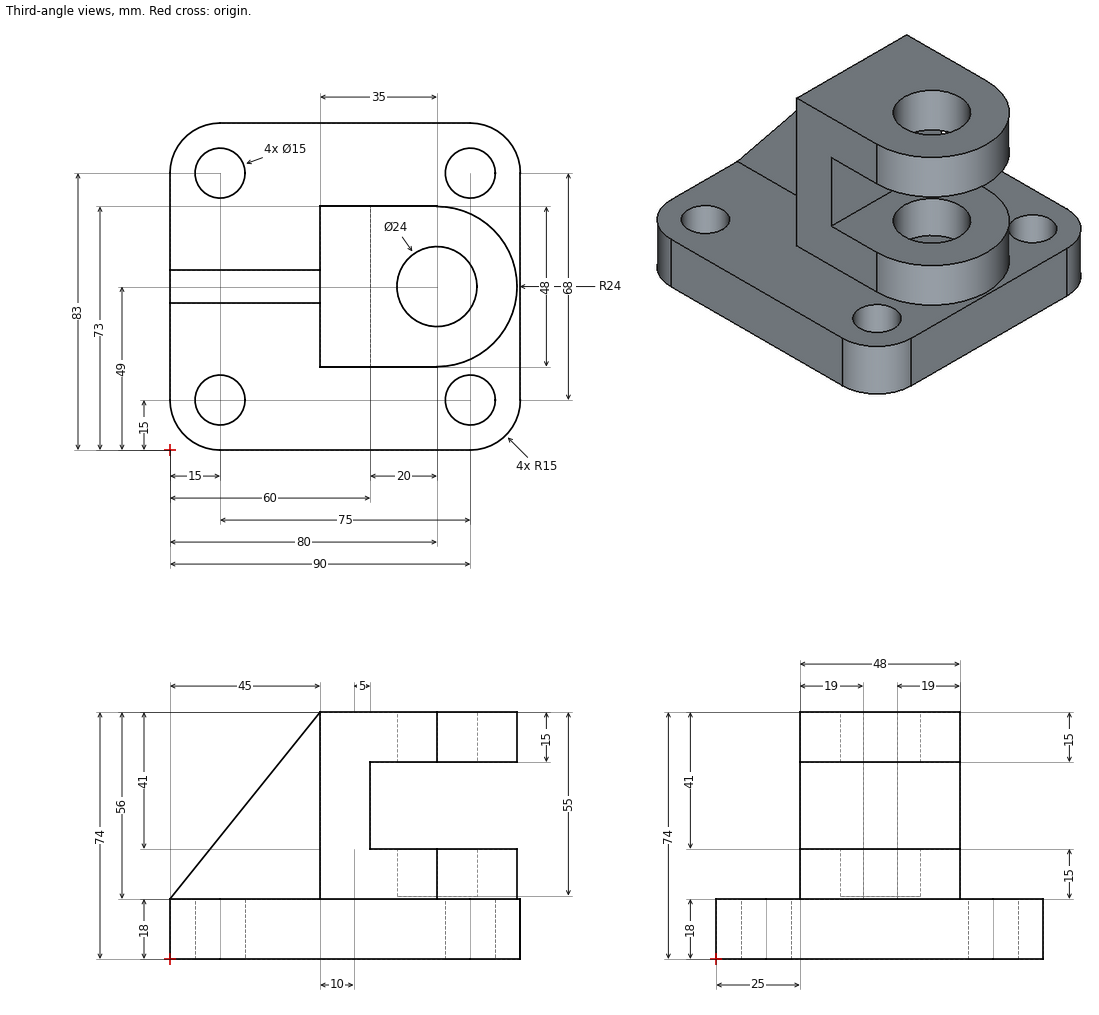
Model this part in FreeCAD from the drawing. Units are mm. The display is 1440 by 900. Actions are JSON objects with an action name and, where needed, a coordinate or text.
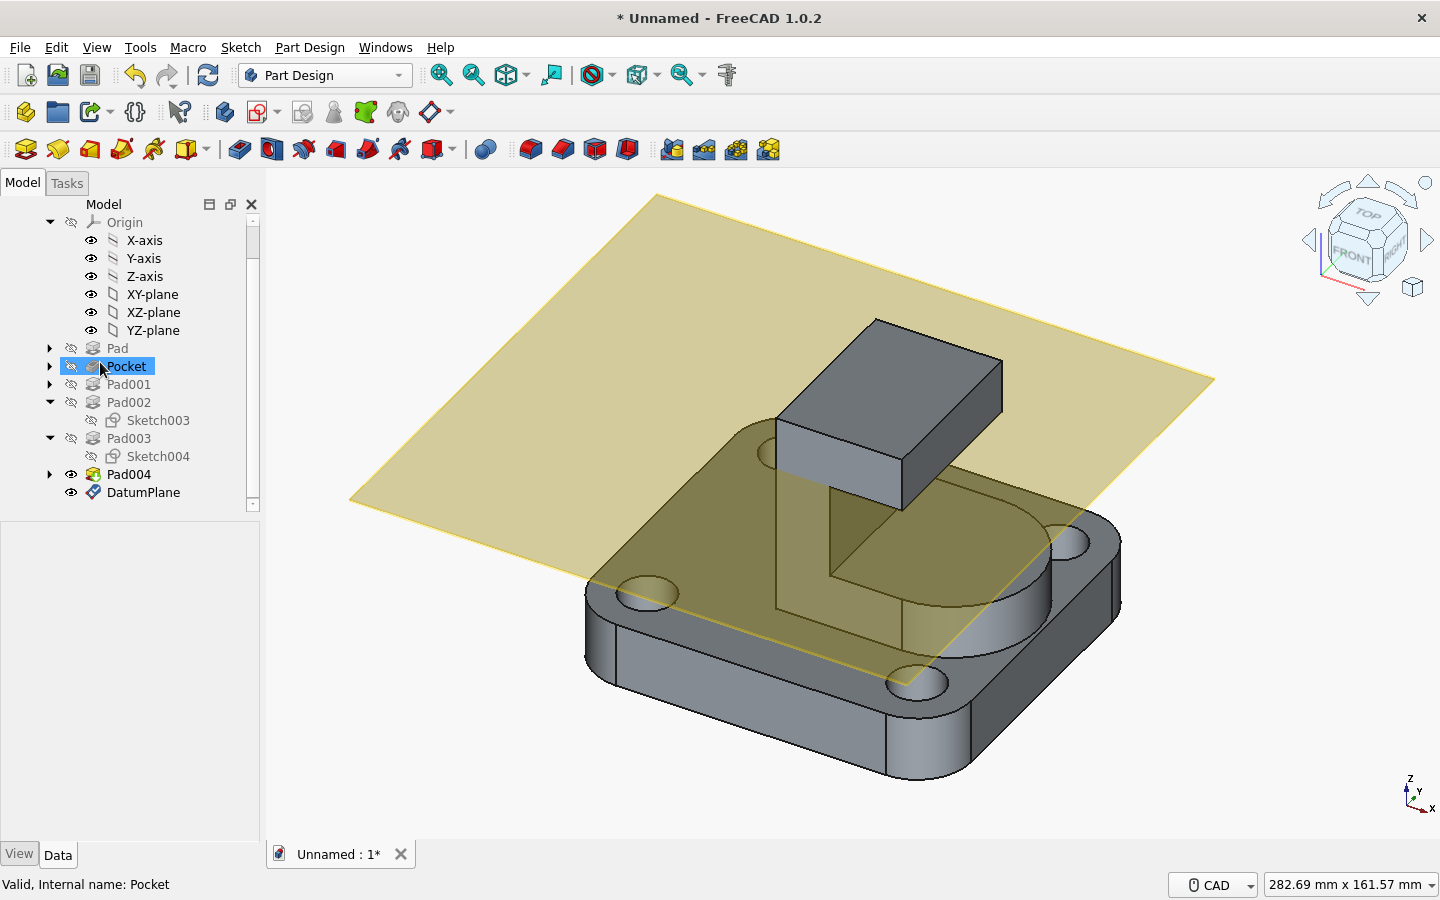
{"action": "left_click", "coordinate": [116, 492]}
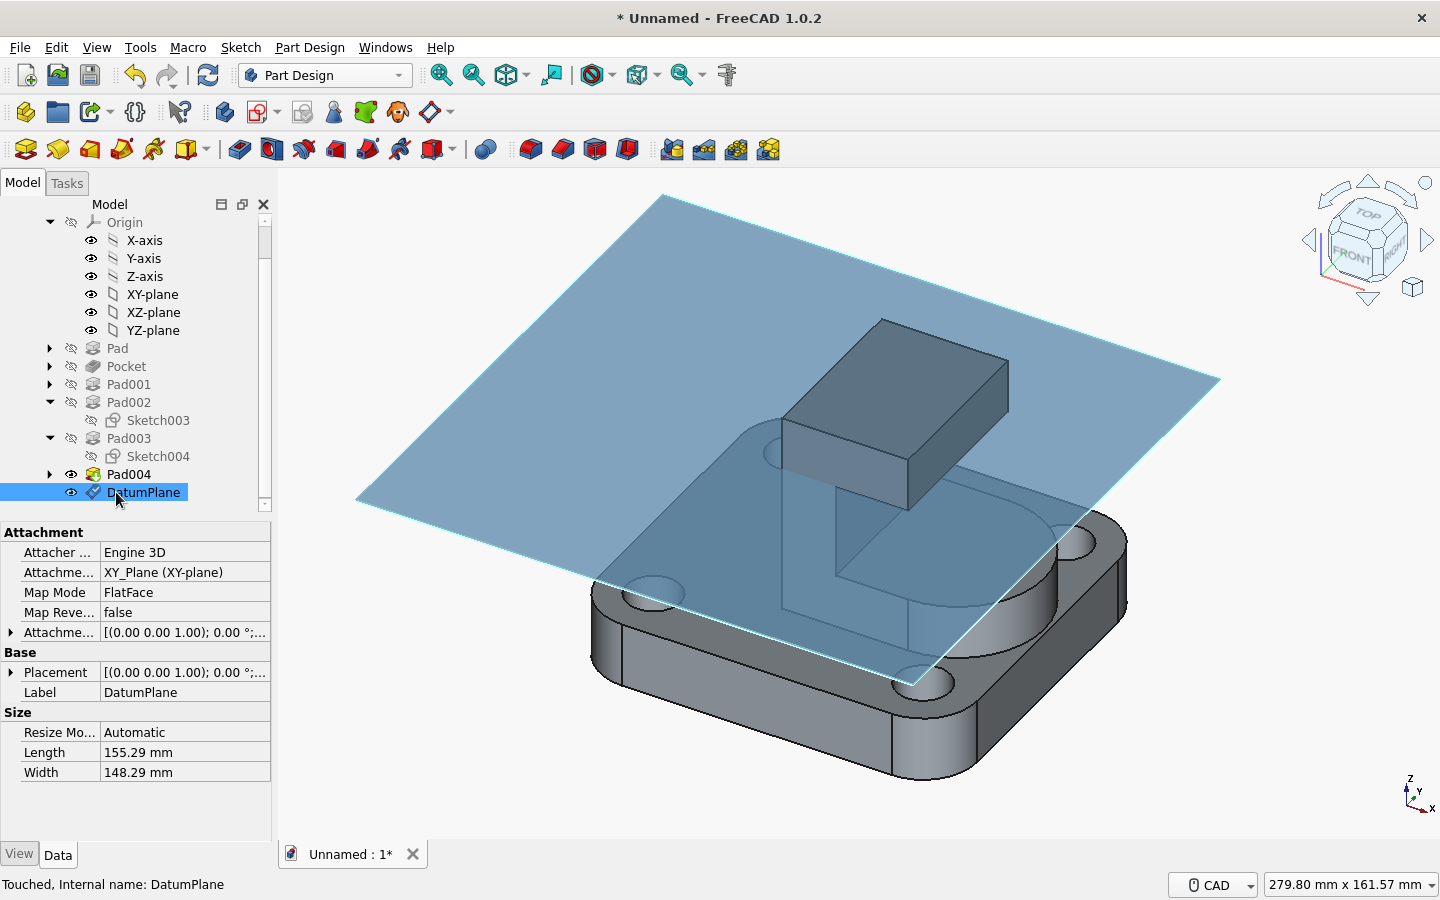
{"action": "left_click", "coordinate": [258, 112]}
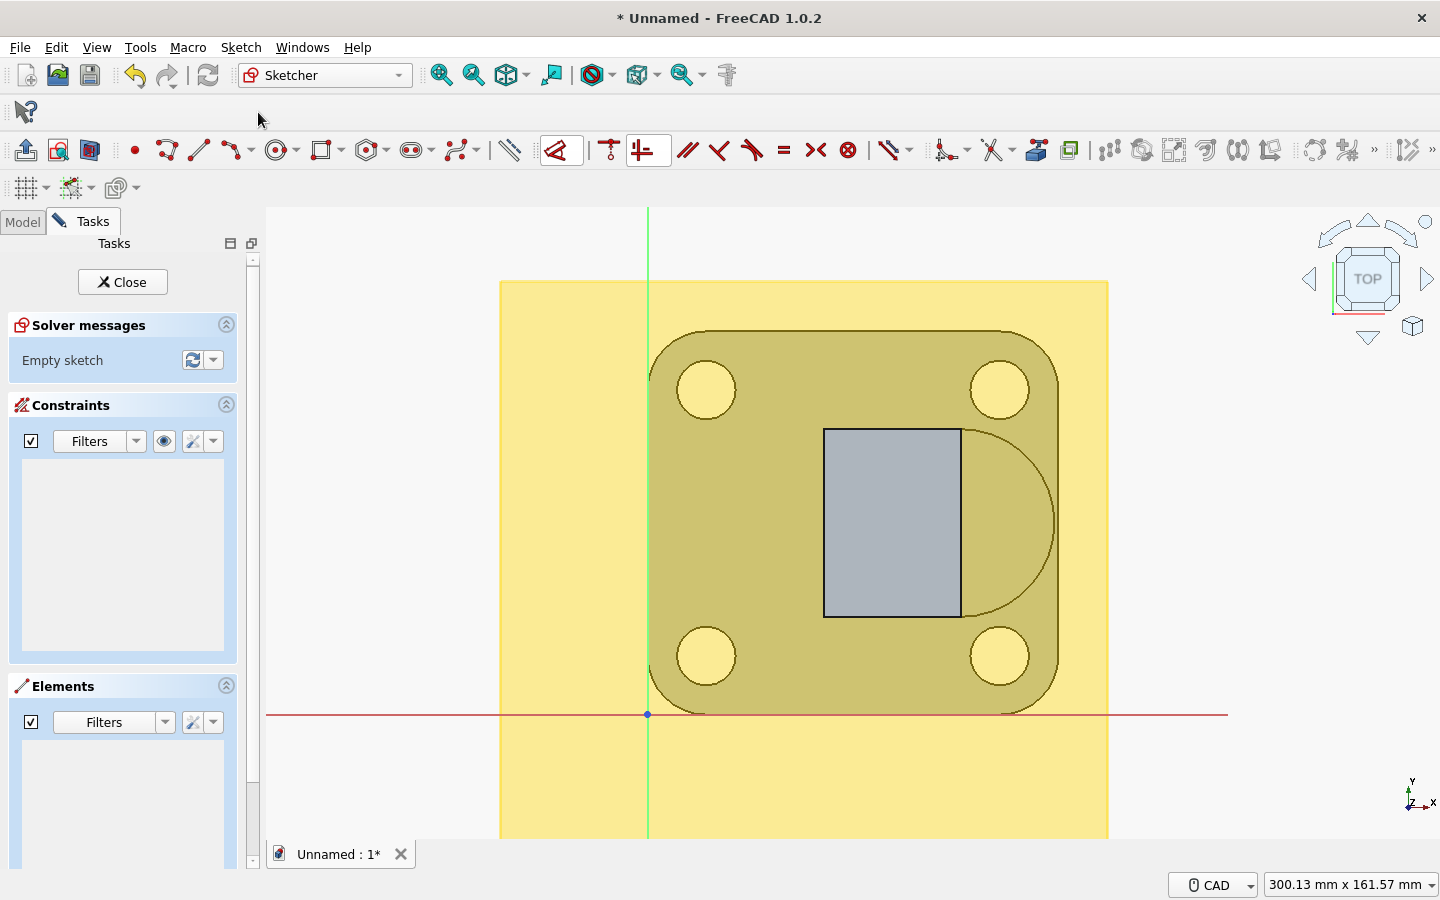
{"action": "left_click", "coordinate": [90, 150]}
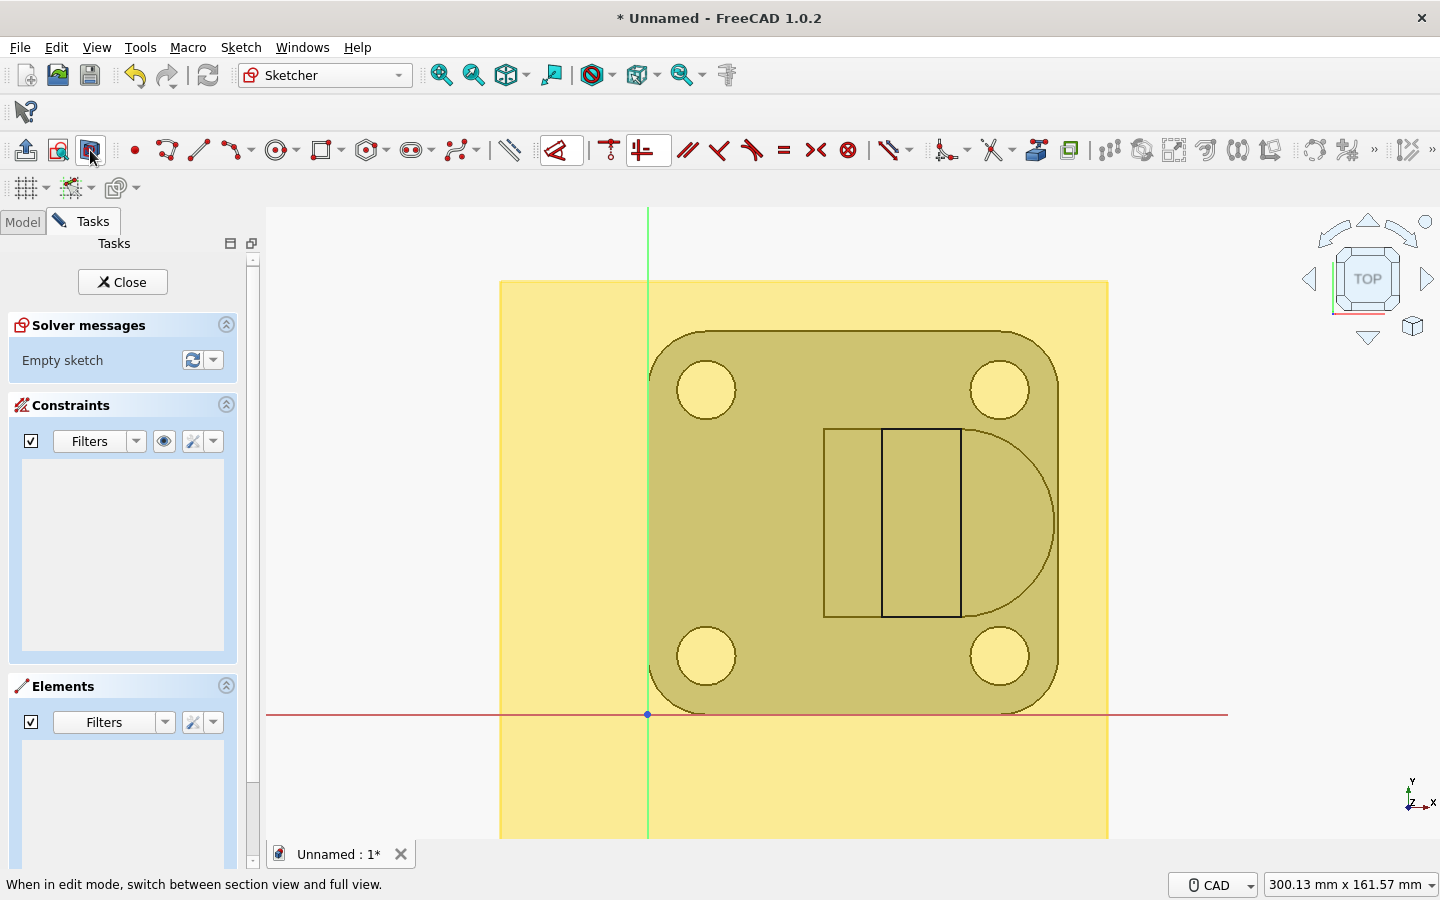
{"action": "scroll", "coordinate": [986, 671], "scroll_direction": "up", "scroll_amount": 2}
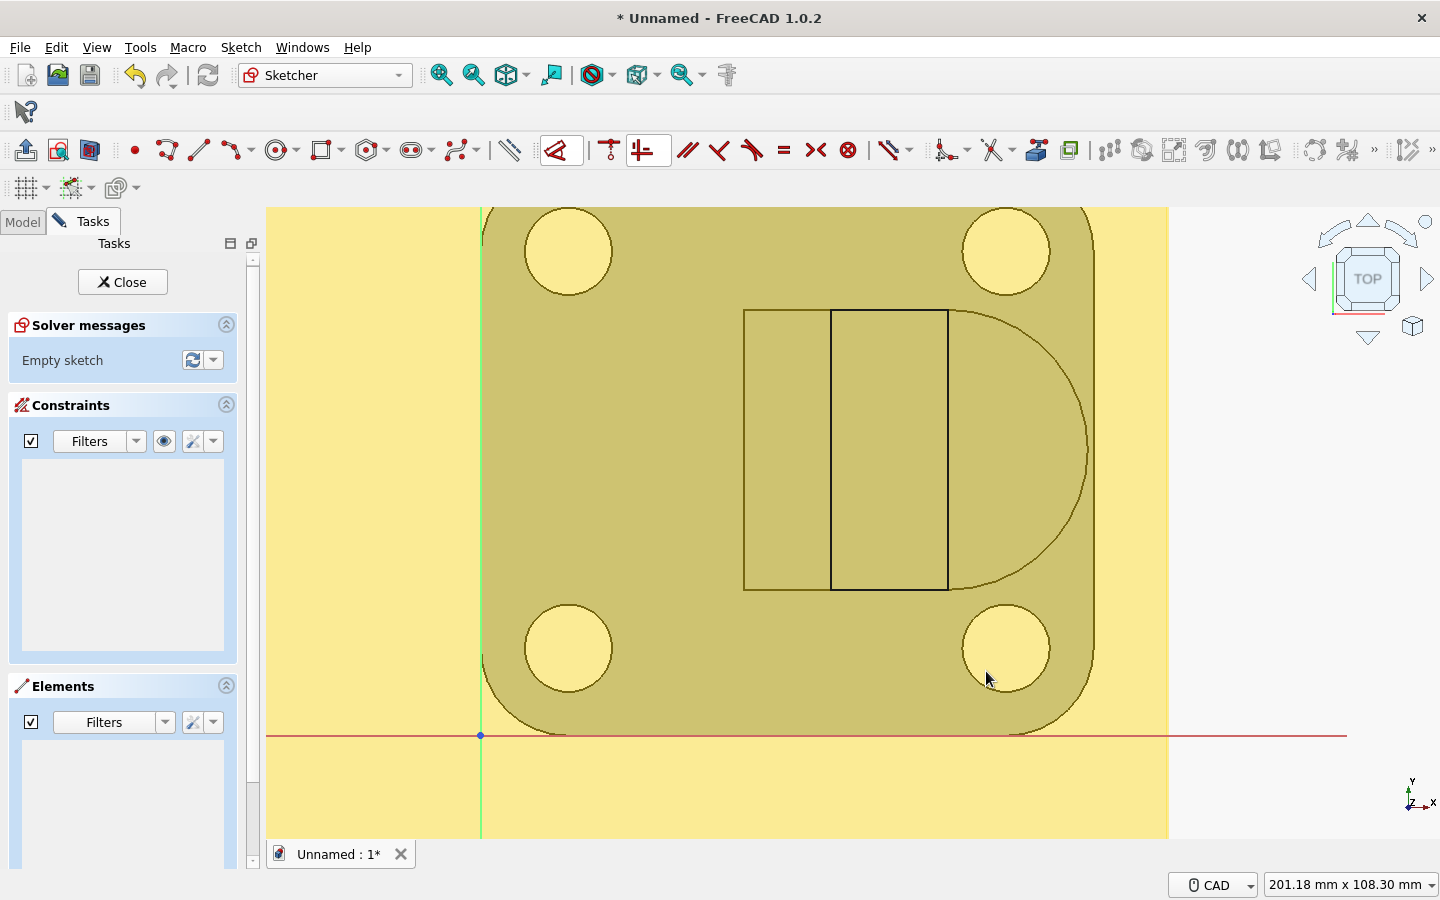
{"action": "left_click", "coordinate": [200, 150]}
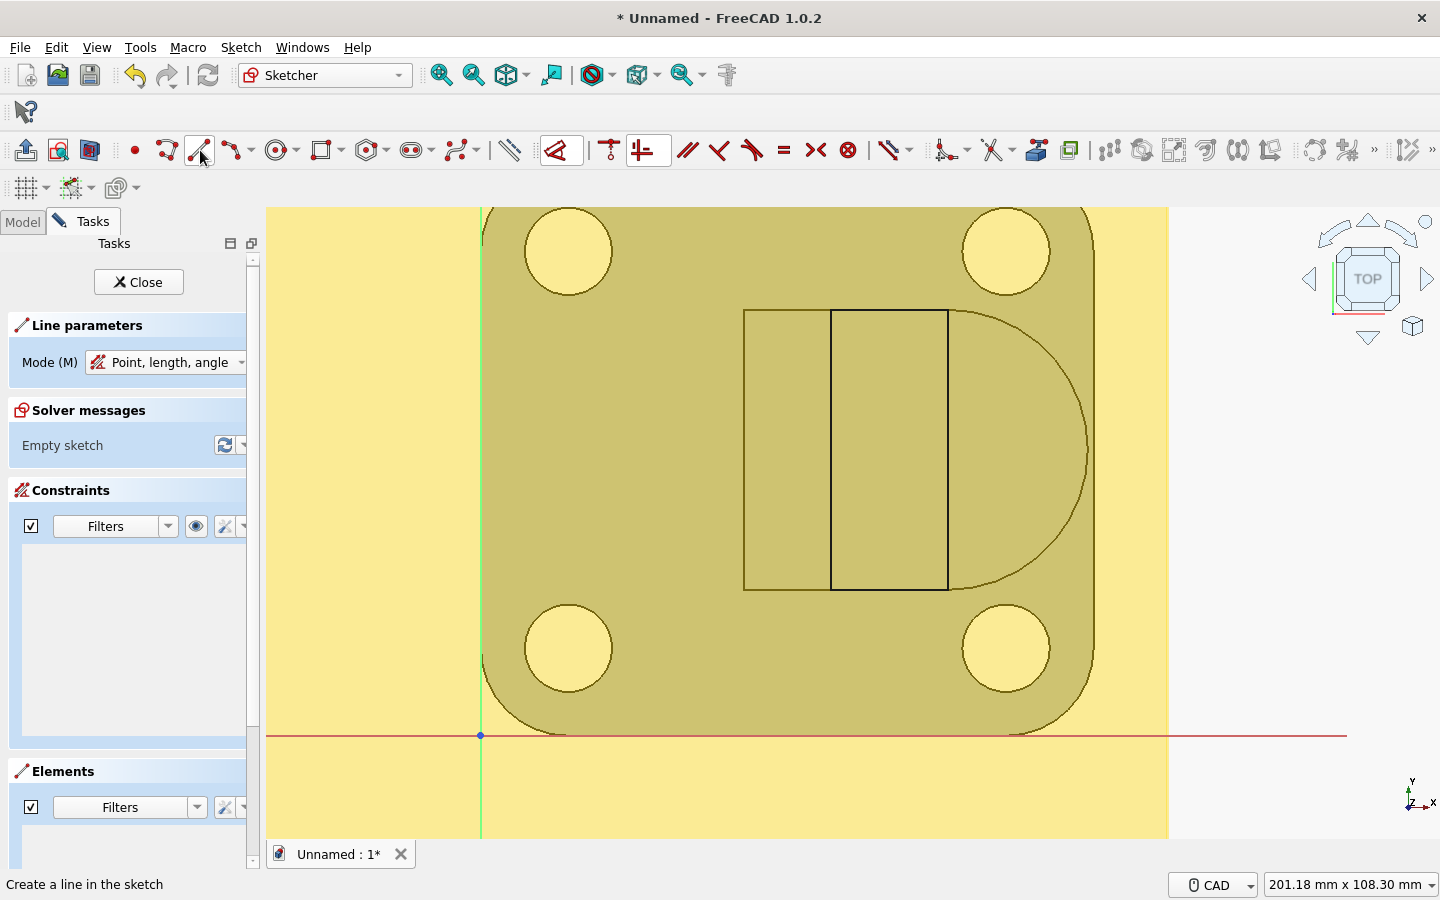
{"action": "left_click", "coordinate": [948, 310]}
{"action": "left_click", "coordinate": [948, 590]}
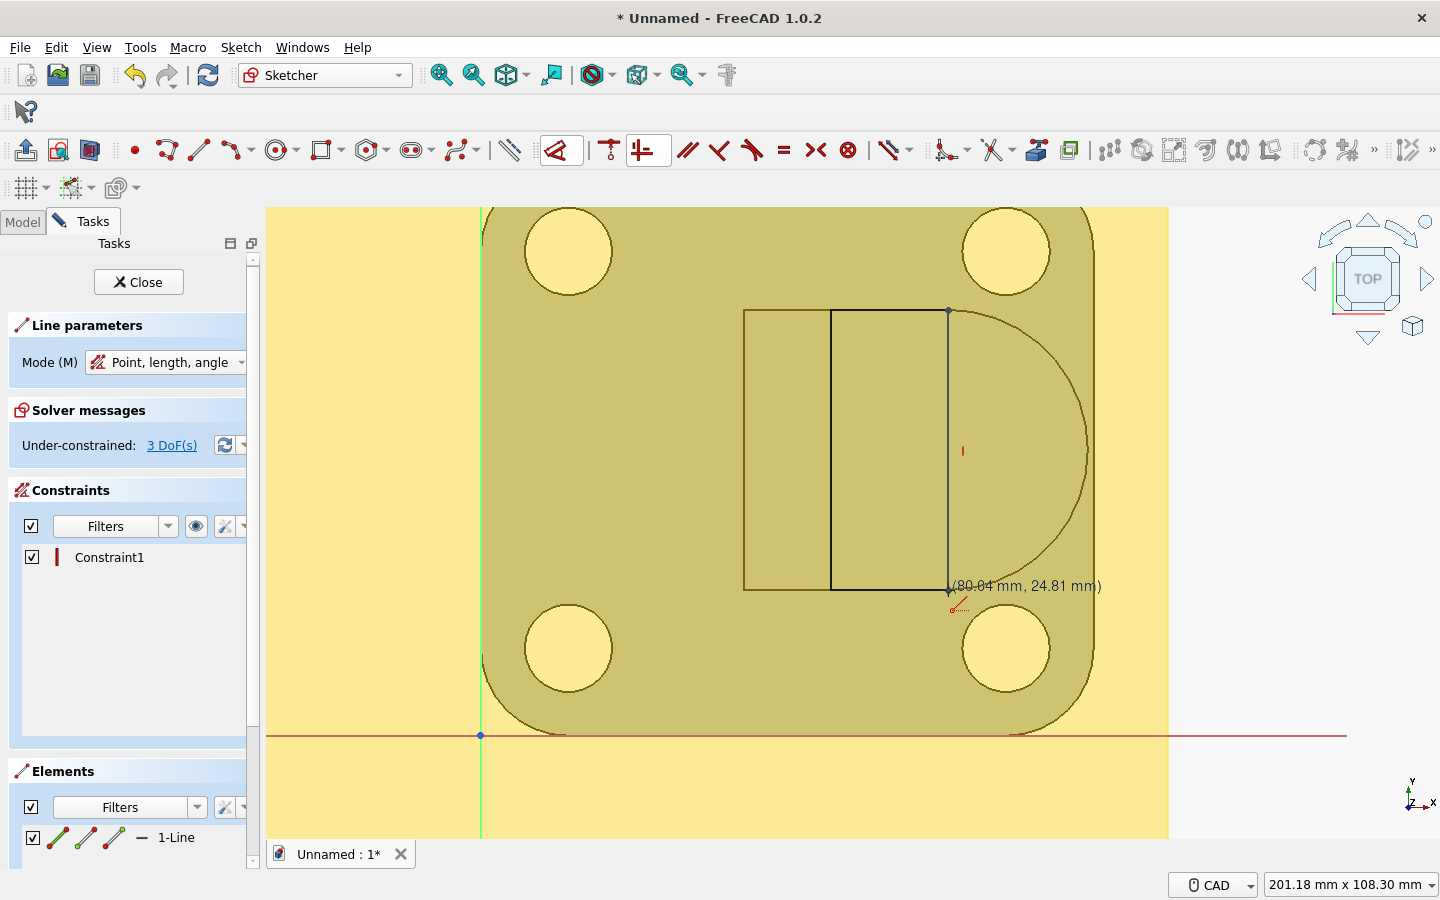
{"action": "left_click", "coordinate": [232, 150]}